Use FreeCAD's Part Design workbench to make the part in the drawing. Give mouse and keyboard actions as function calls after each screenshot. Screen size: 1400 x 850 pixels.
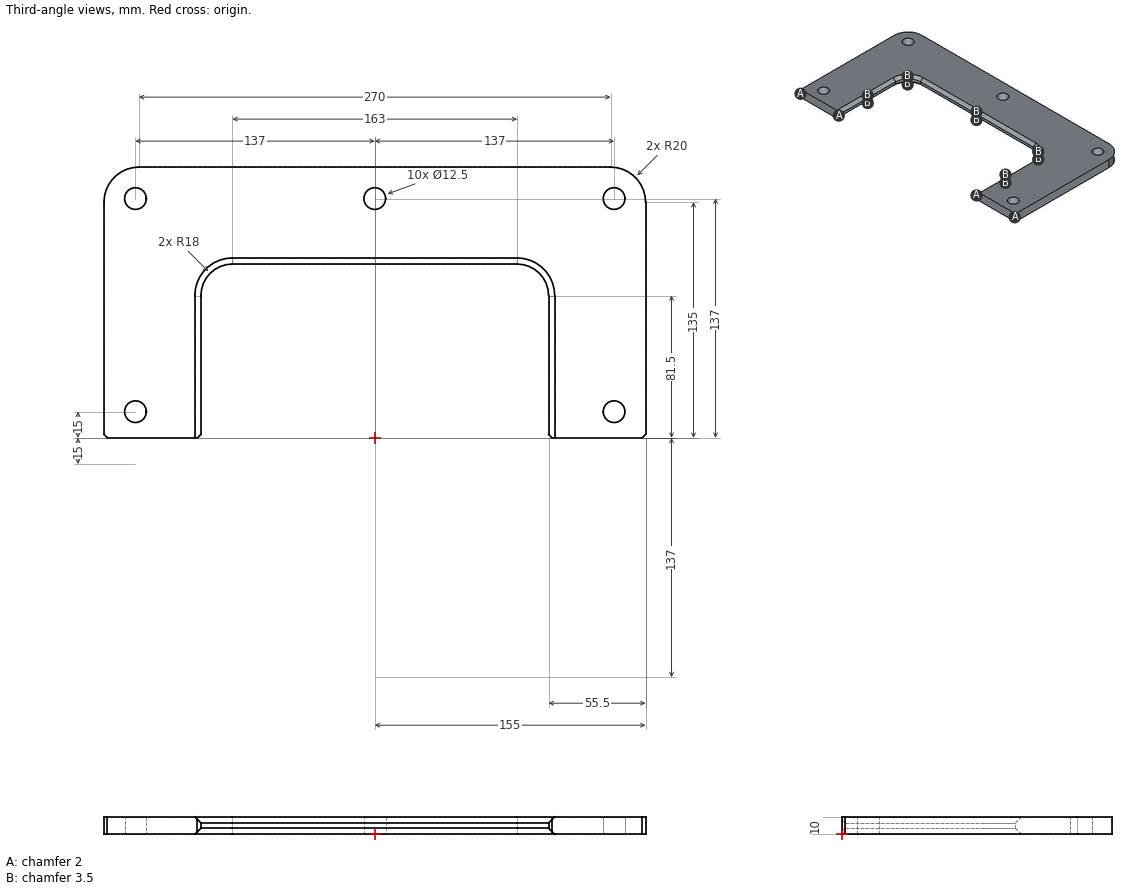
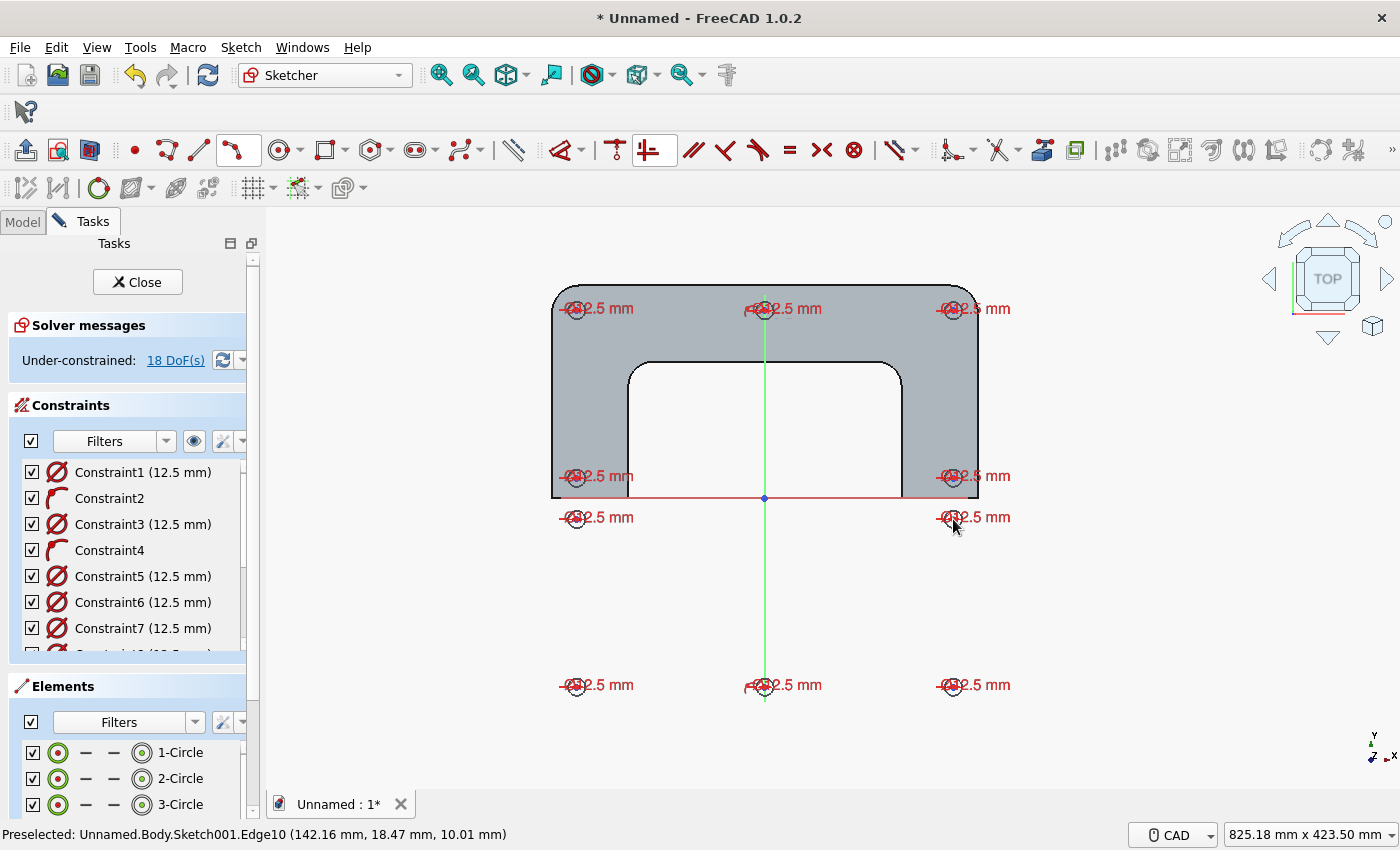
scroll(577, 478, up, 4)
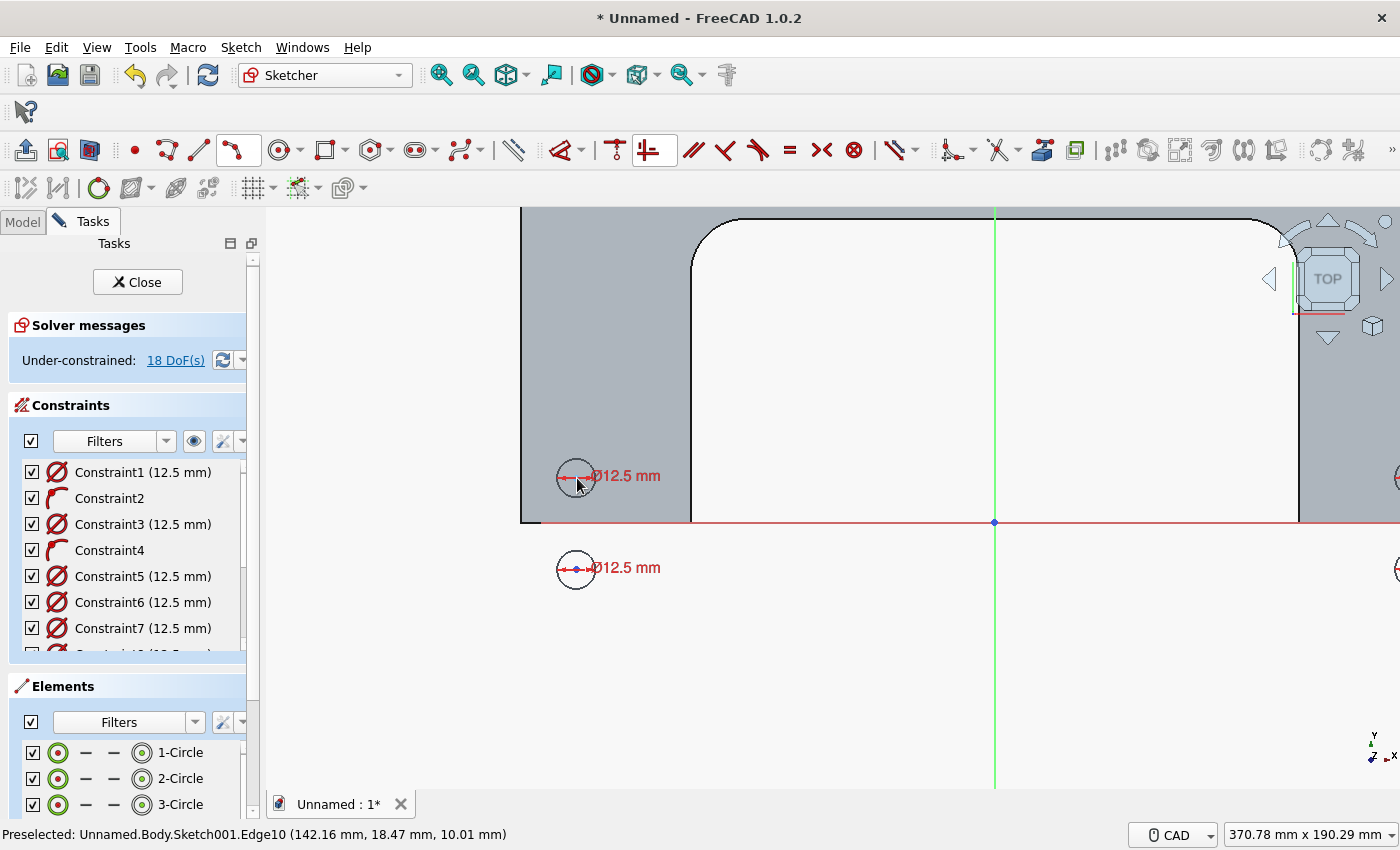
click(576, 478)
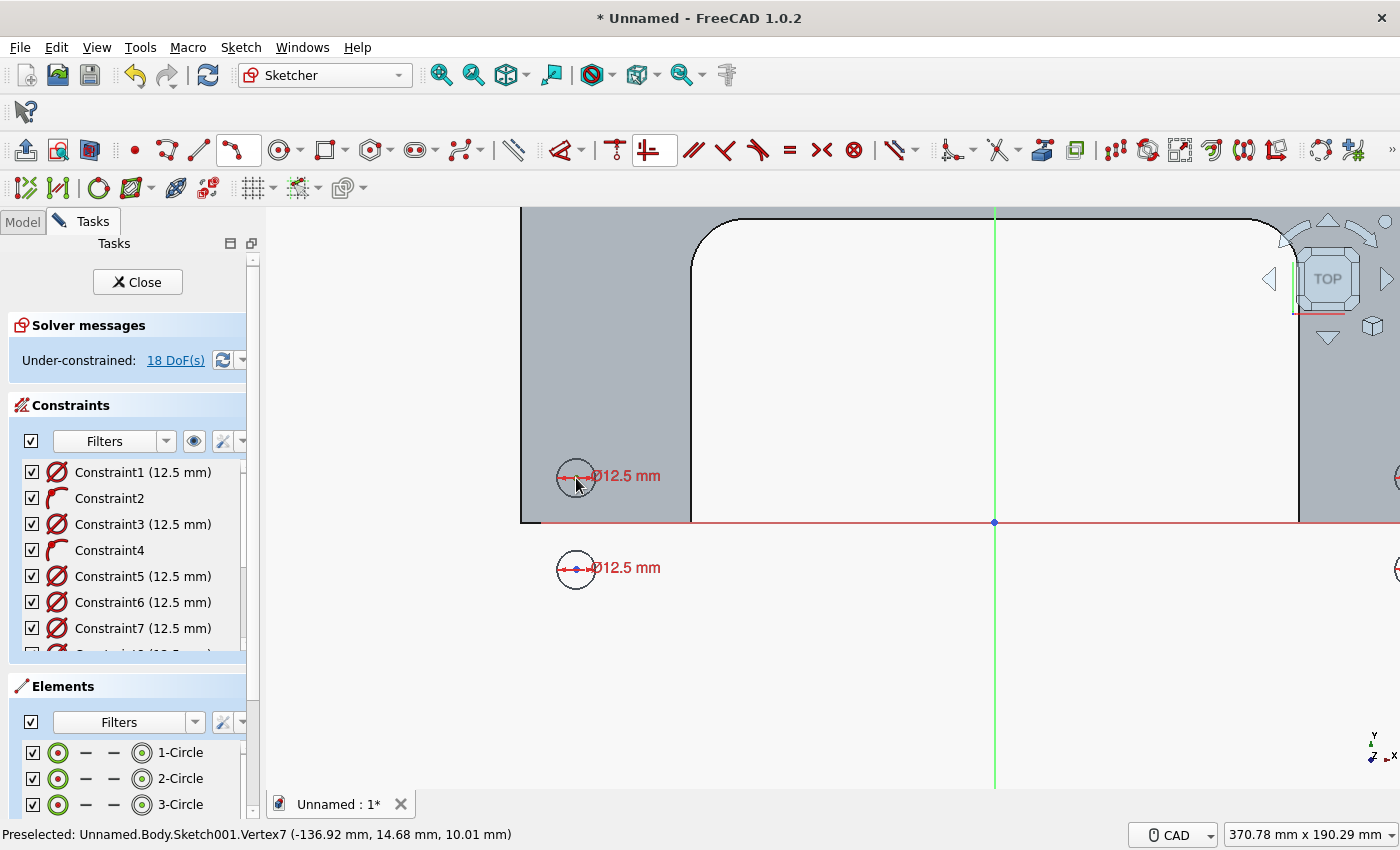
key(i)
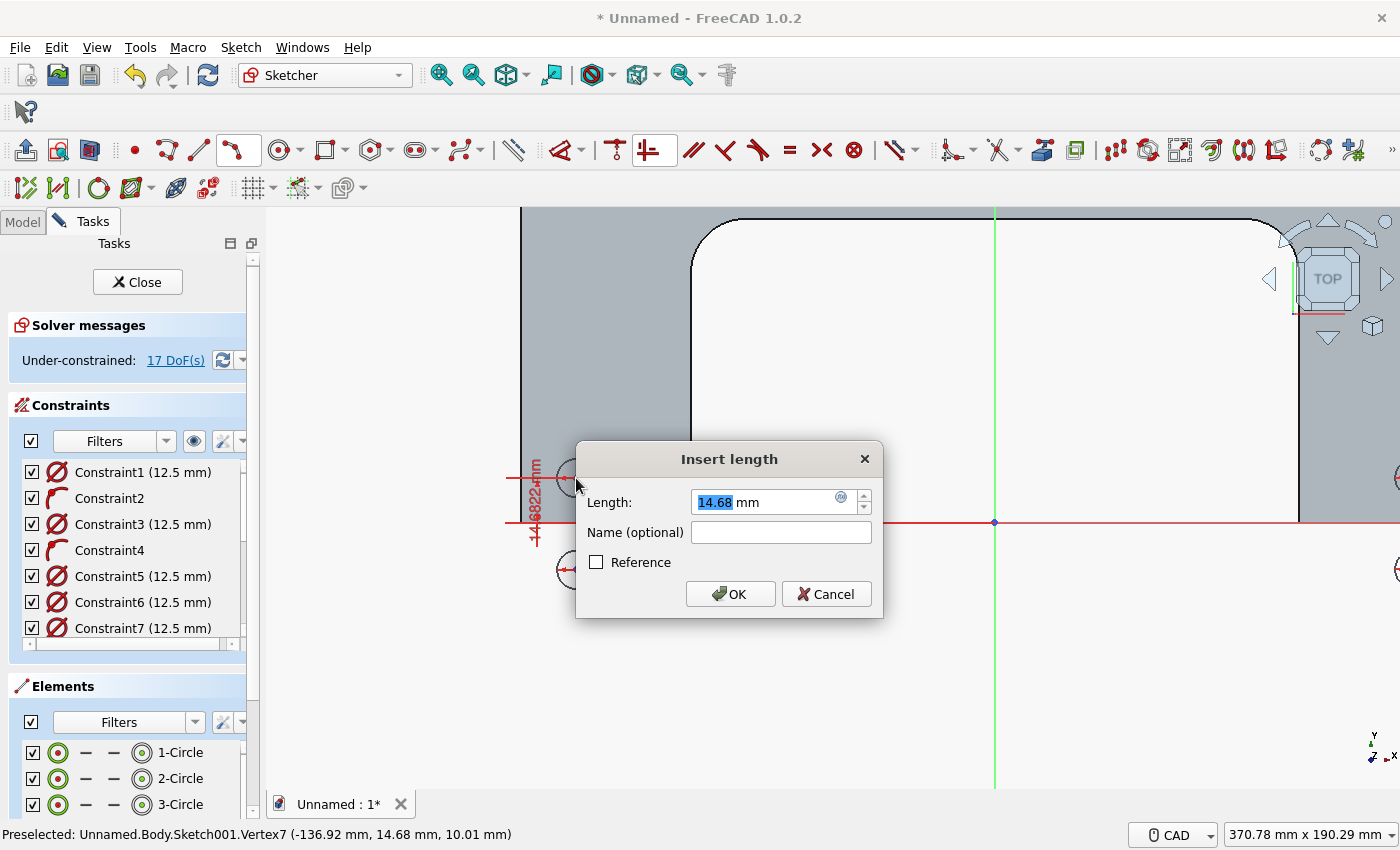
text(15)
key(Return)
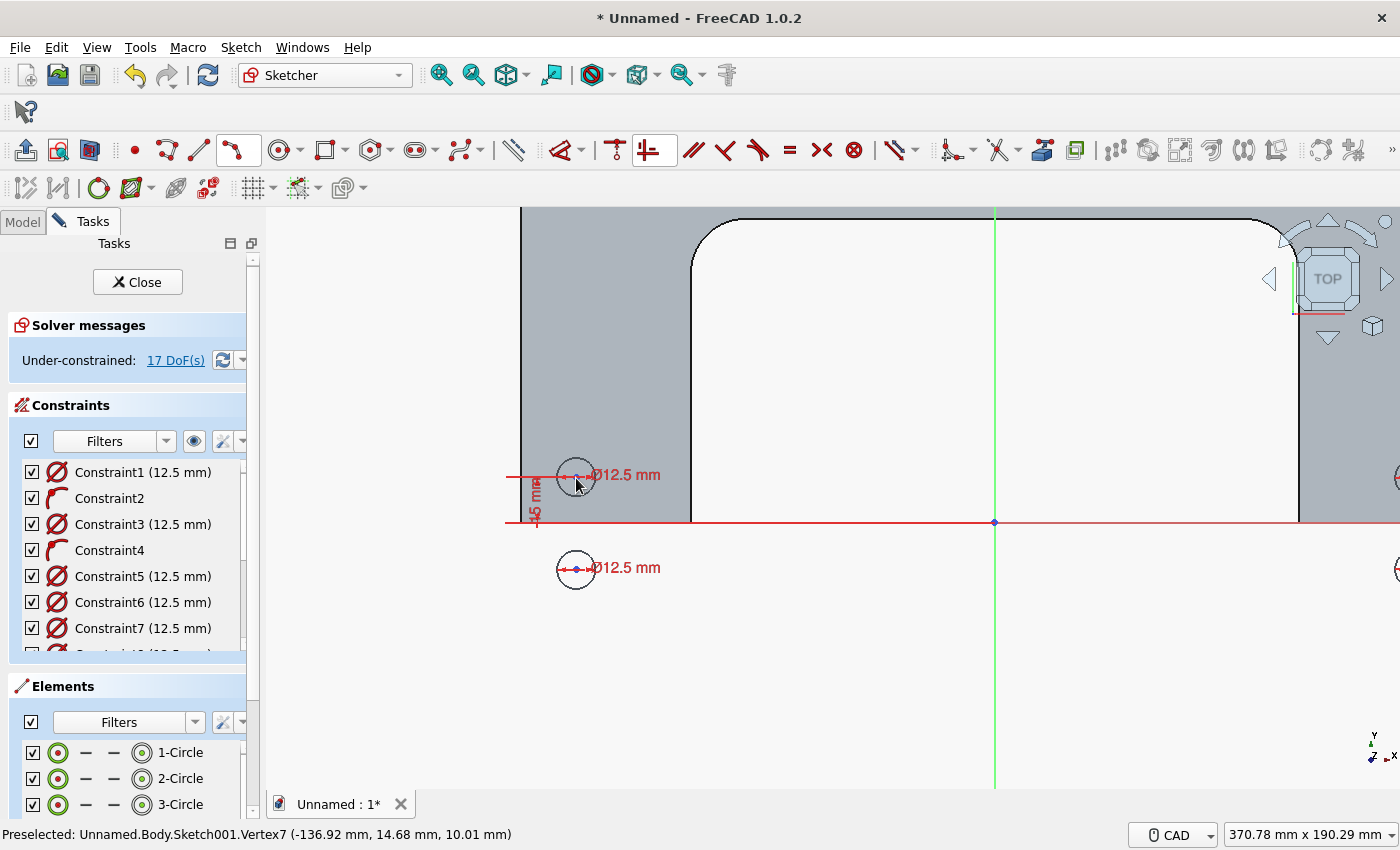
click(576, 570)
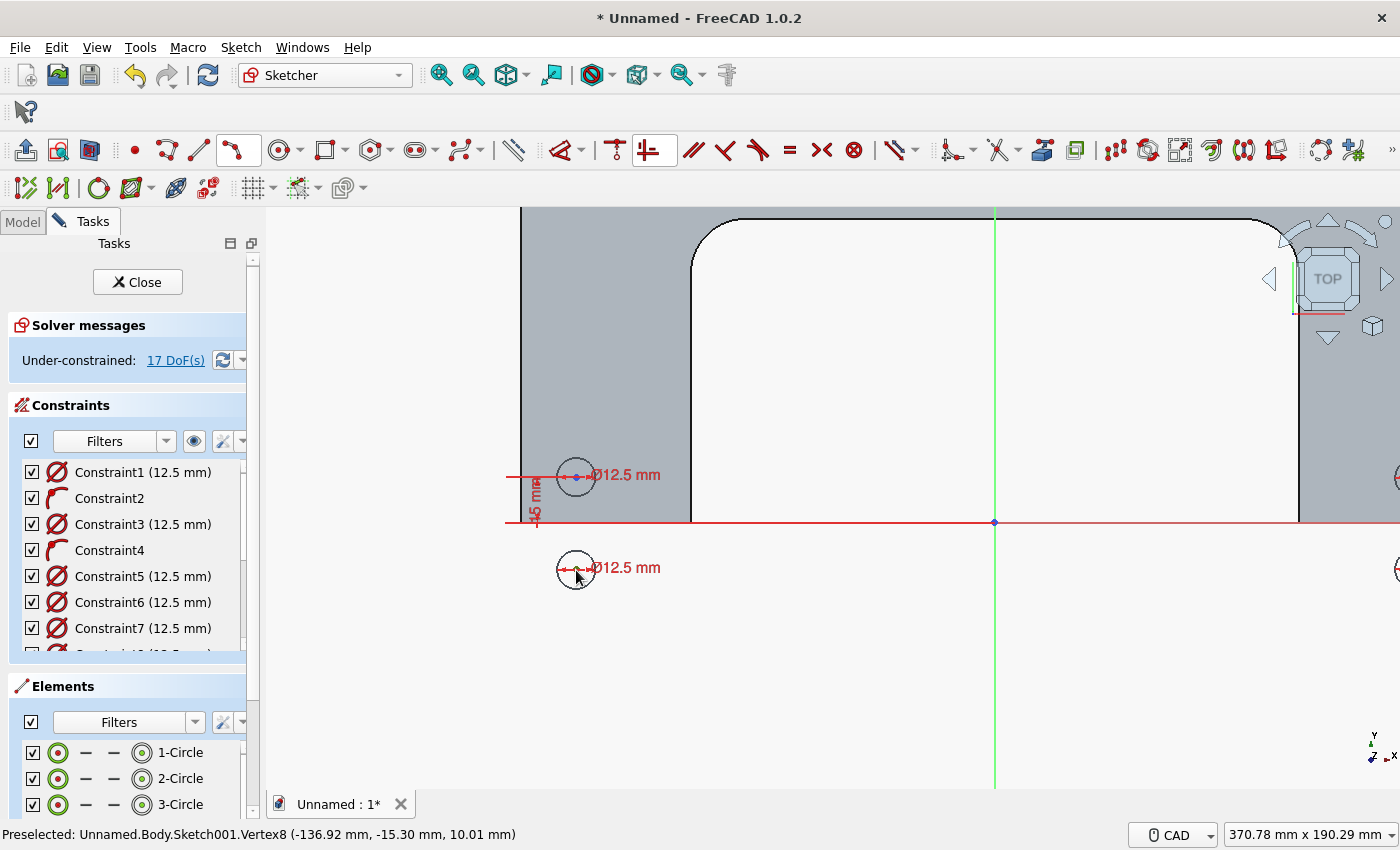
click(584, 150)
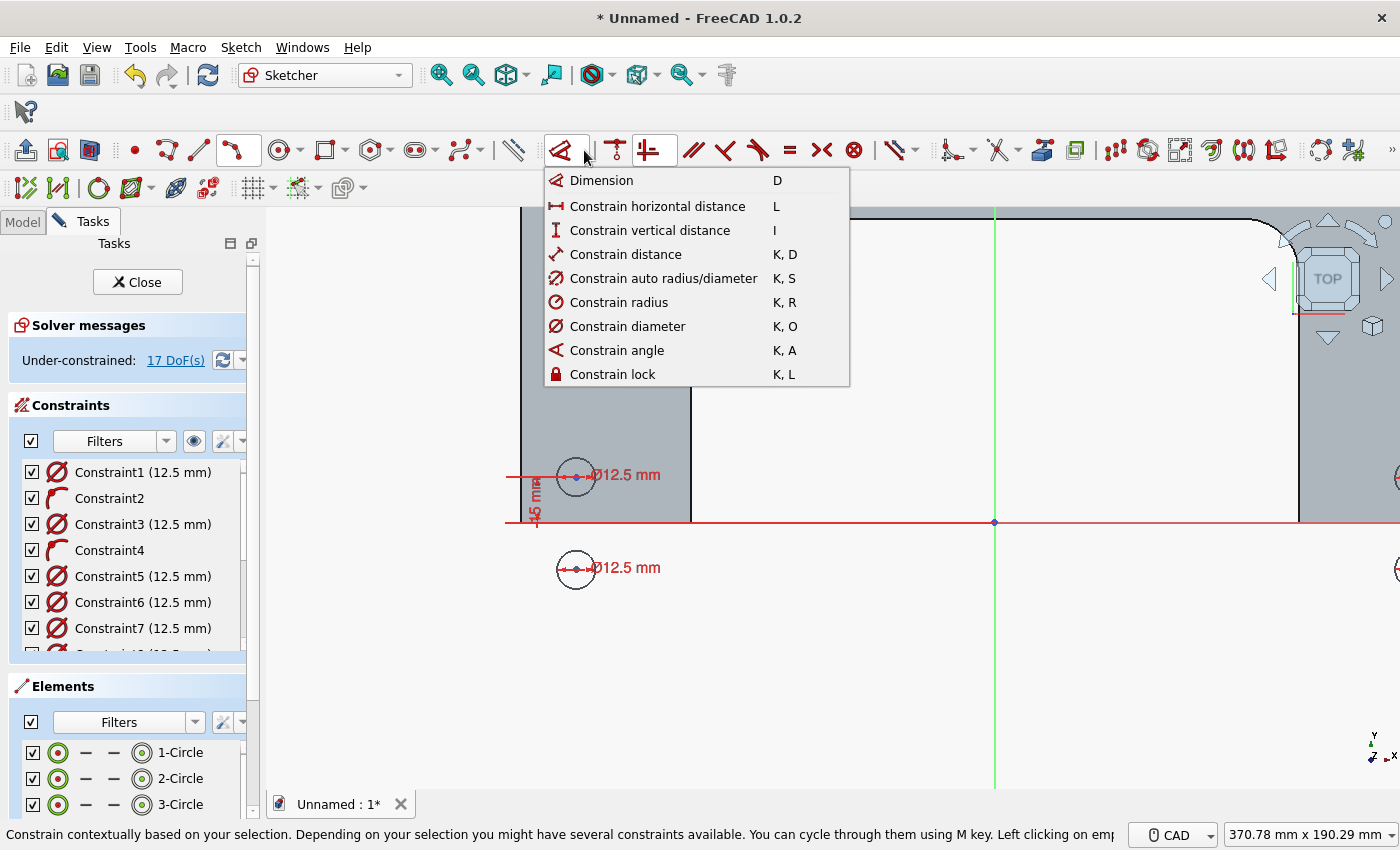
click(697, 230)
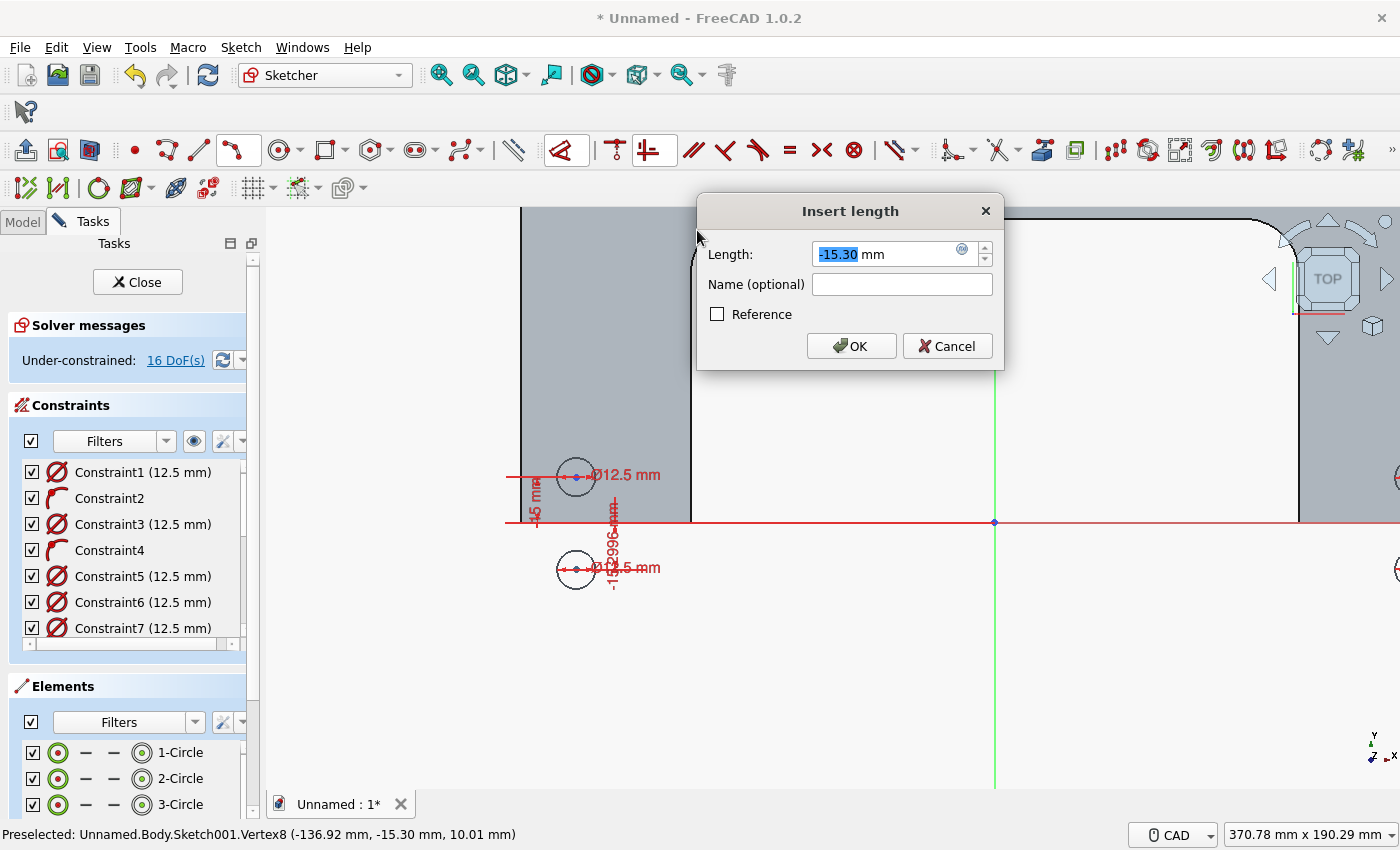
text(-15)
key(Return)